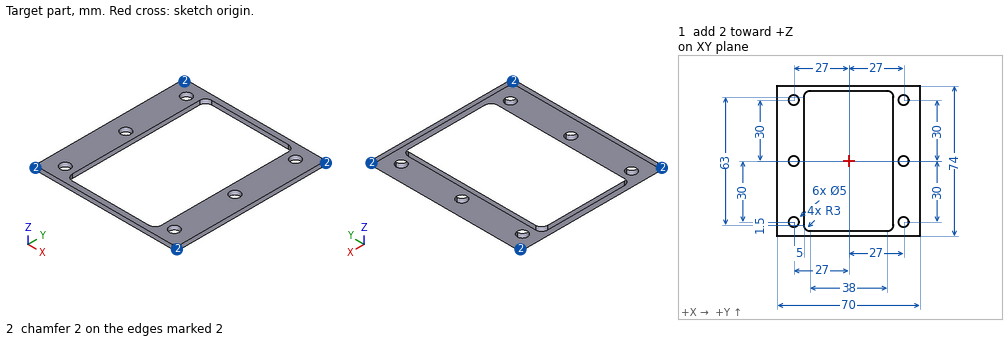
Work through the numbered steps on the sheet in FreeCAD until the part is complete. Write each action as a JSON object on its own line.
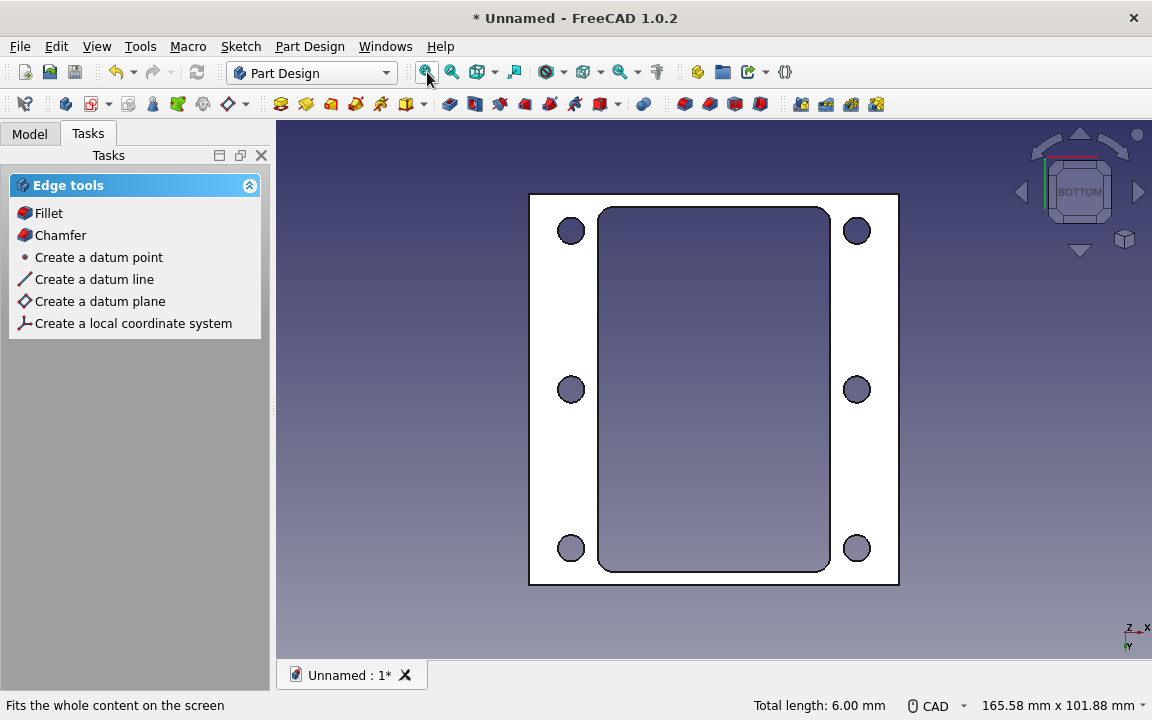
{"action": "scroll", "coordinate": [529, 584], "scroll_direction": "up", "scroll_amount": 7}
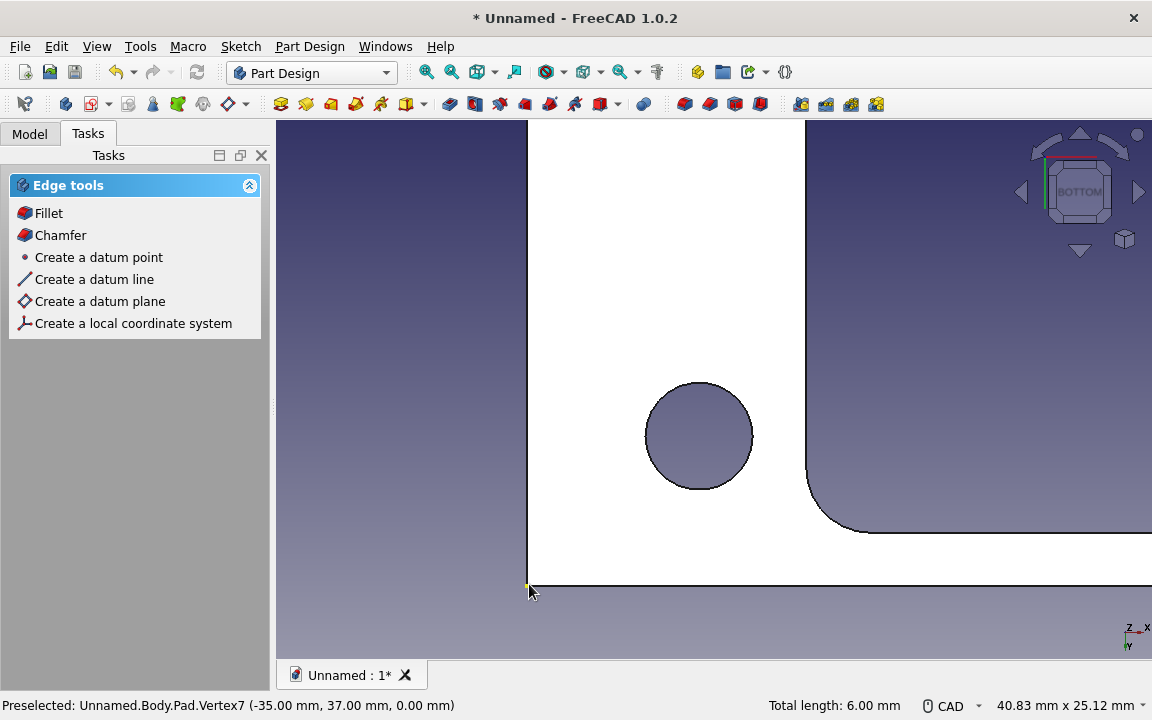
{"action": "left_click", "coordinate": [427, 72]}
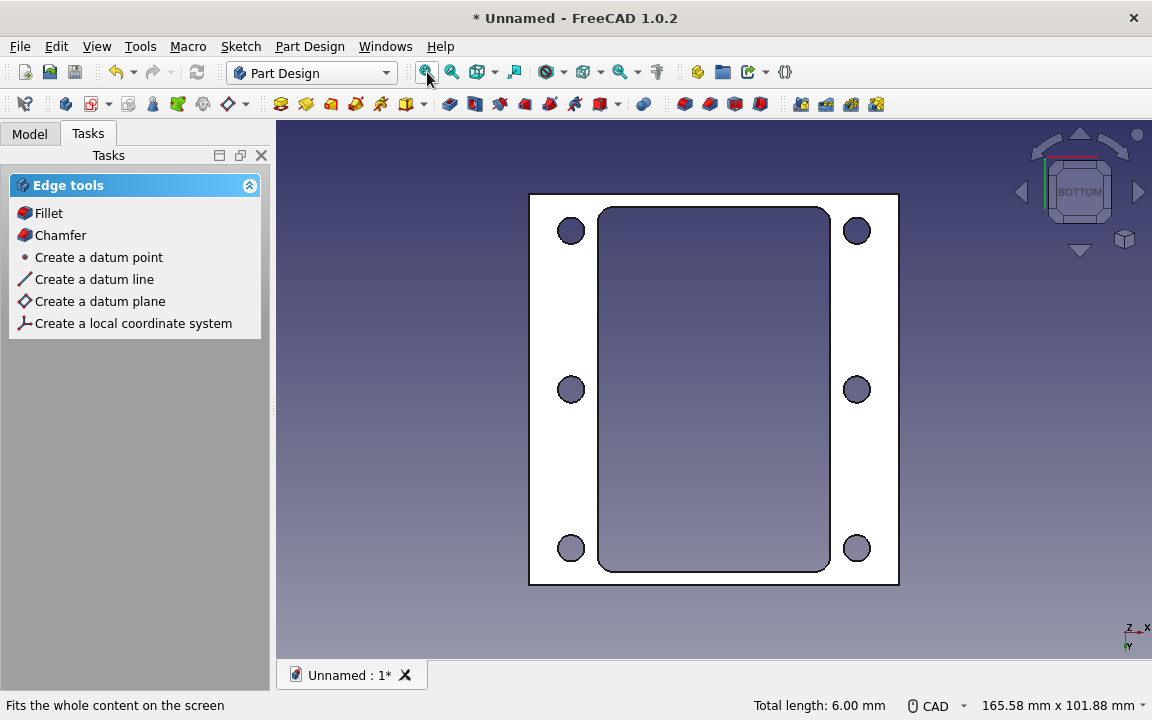
{"action": "key", "text": "4"}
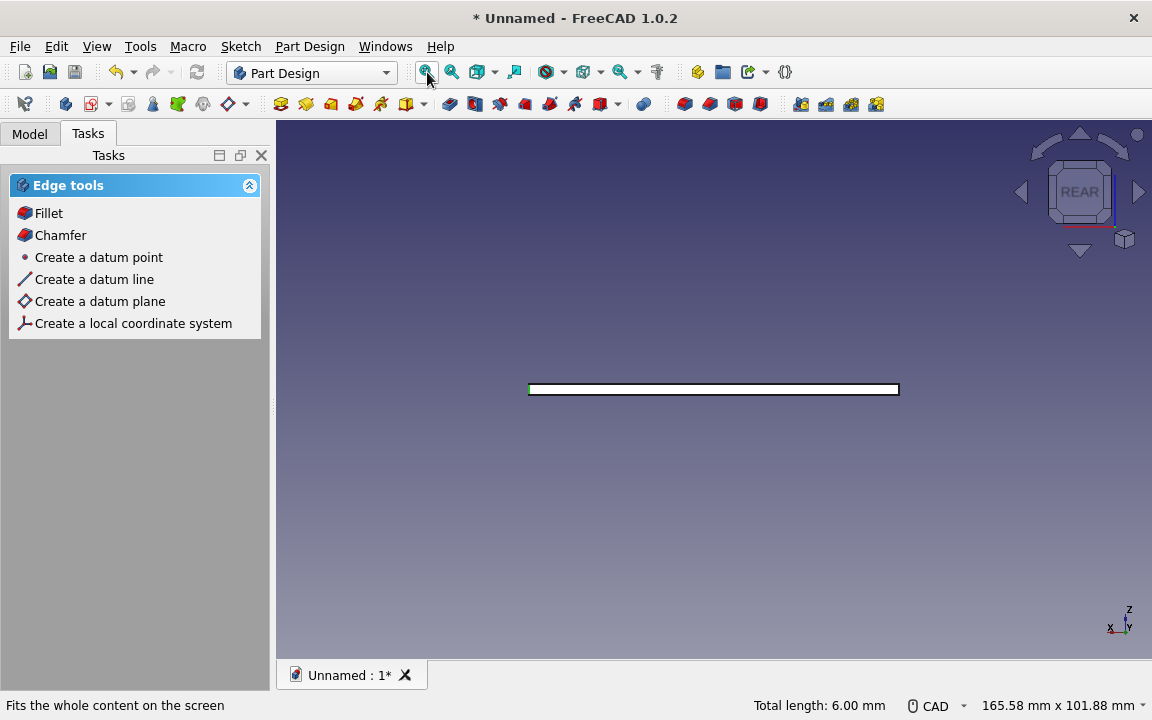
{"action": "left_click", "coordinate": [427, 72]}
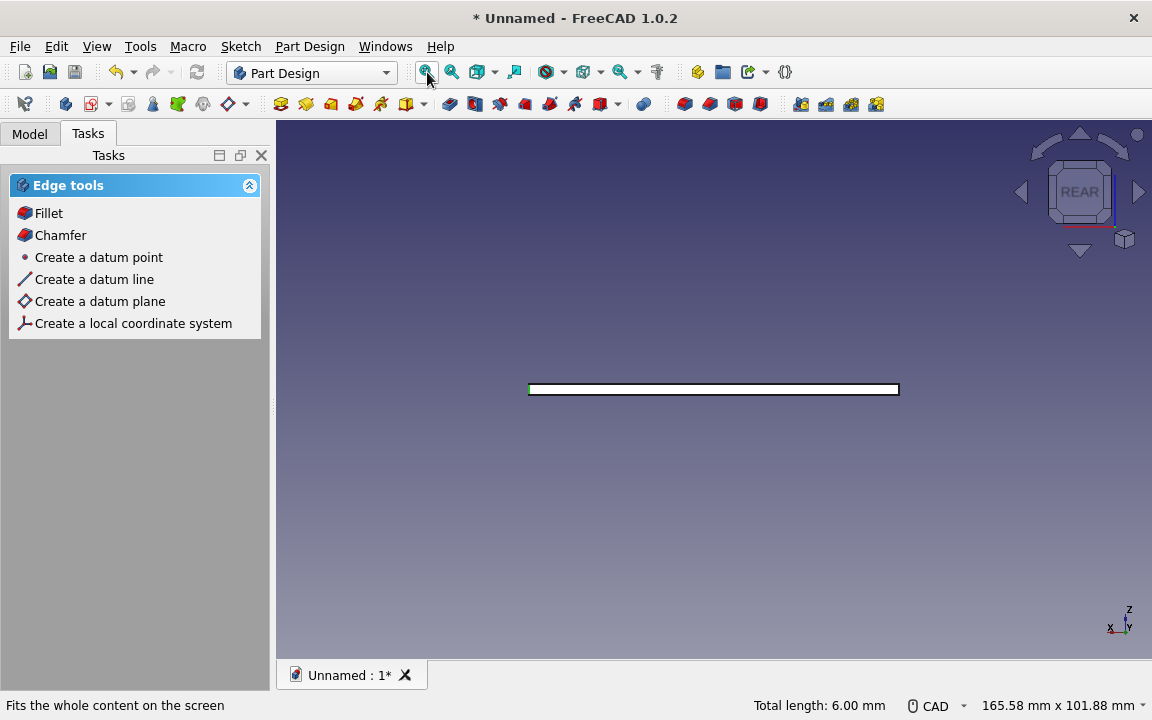
{"action": "scroll", "coordinate": [899, 389], "scroll_direction": "up", "scroll_amount": 7}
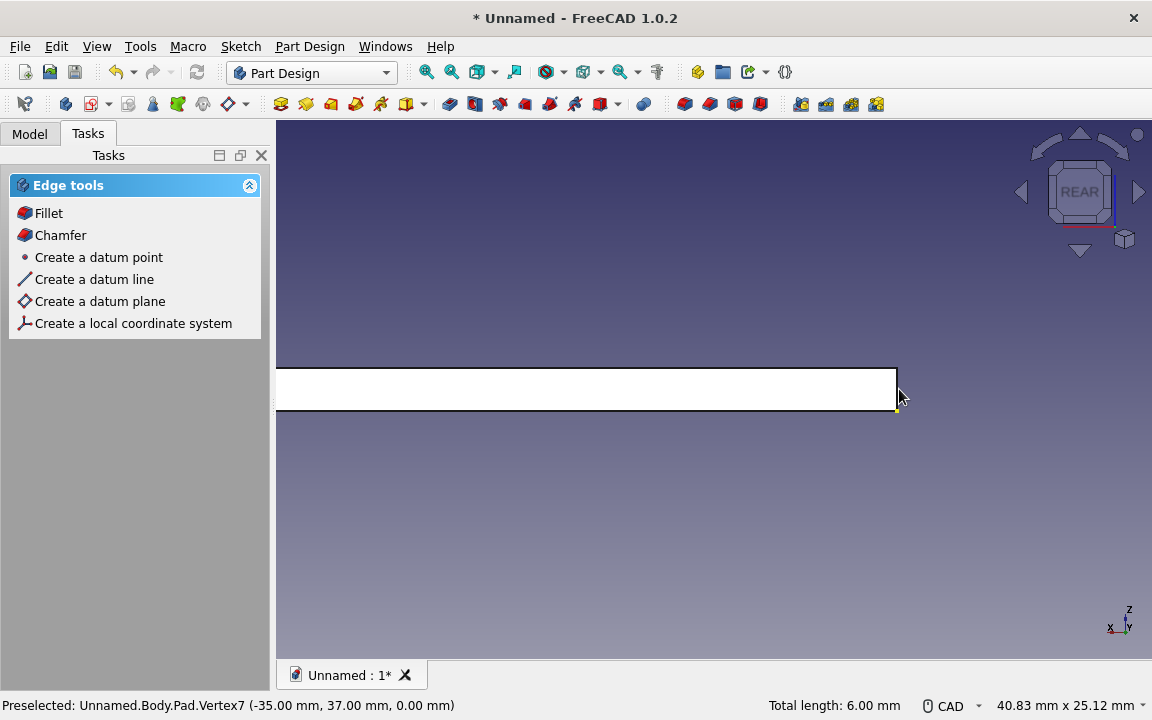
{"action": "left_click", "coordinate": [897, 389], "text": "ctrl"}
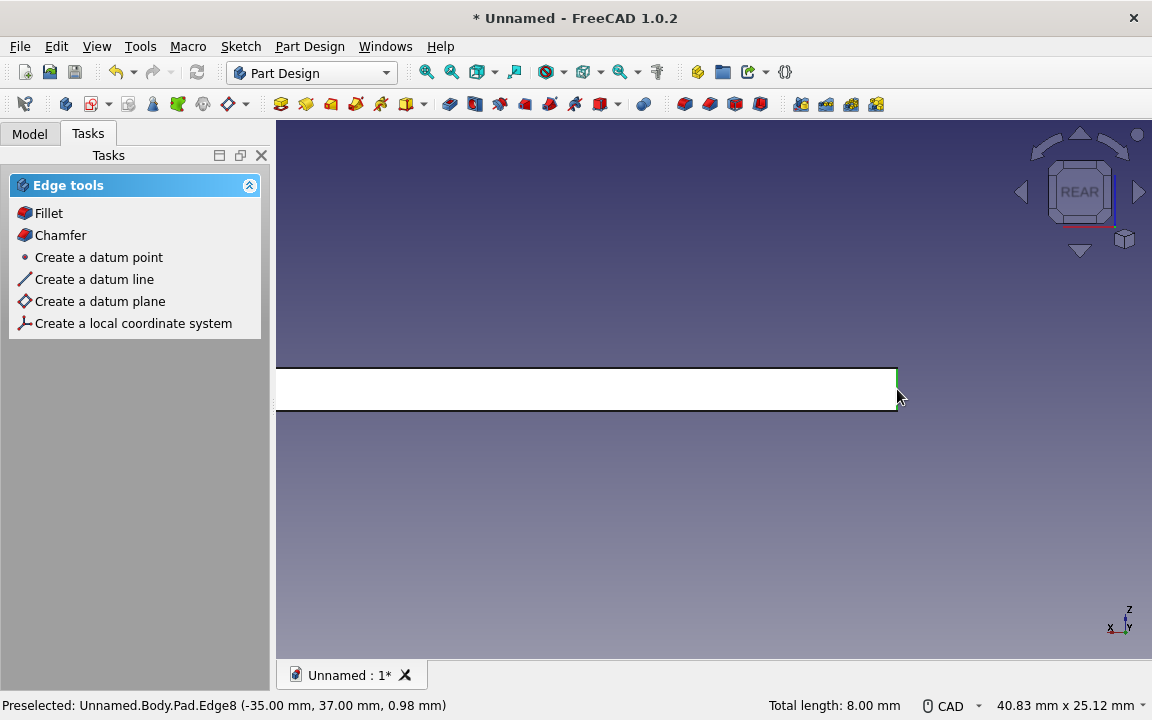
{"action": "left_click", "coordinate": [710, 104]}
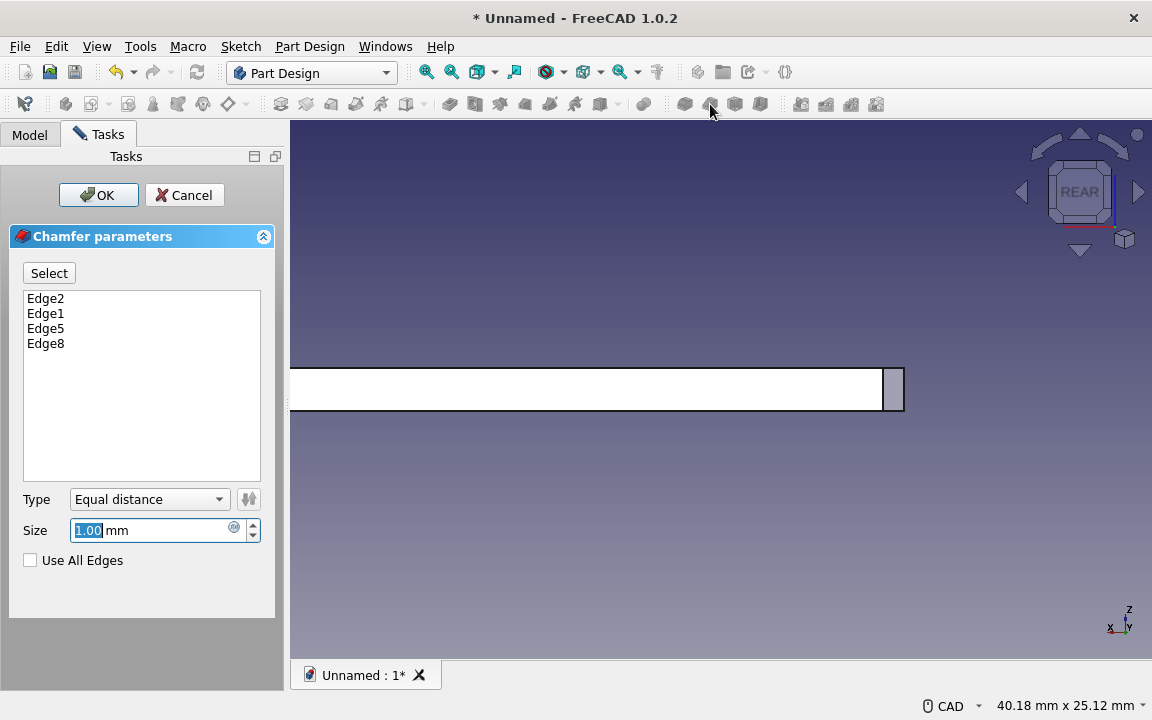
{"action": "type", "text": "2"}
{"action": "key", "text": "Tab"}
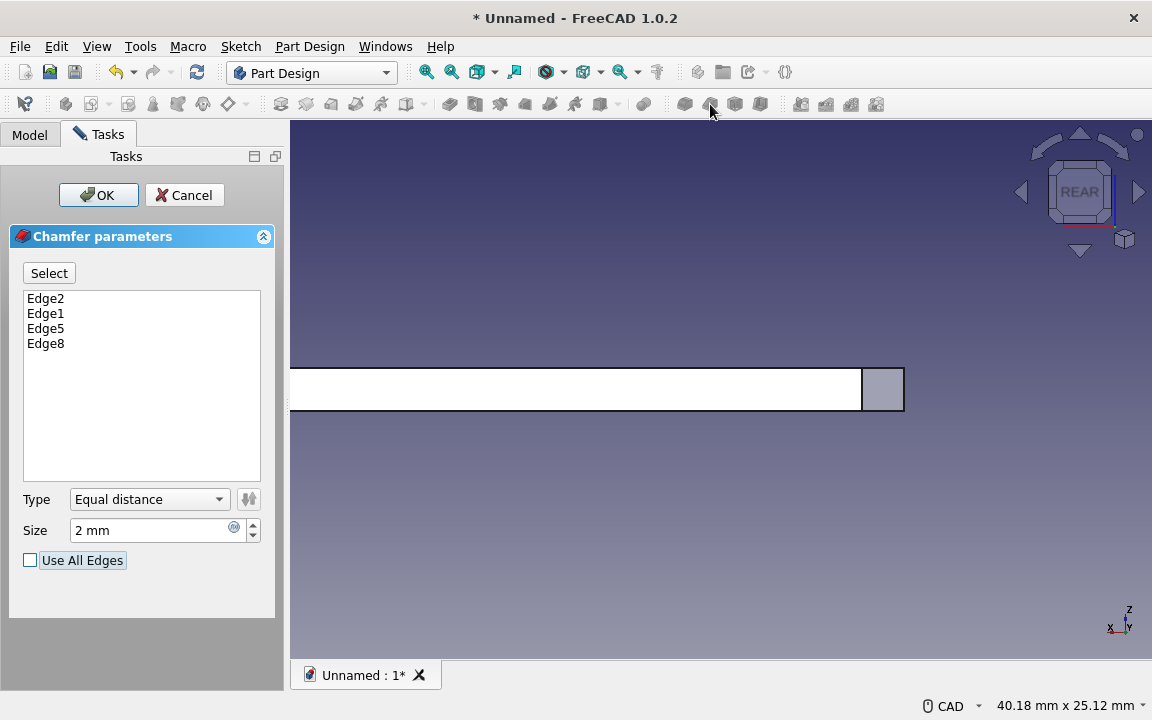
{"action": "left_click", "coordinate": [99, 195]}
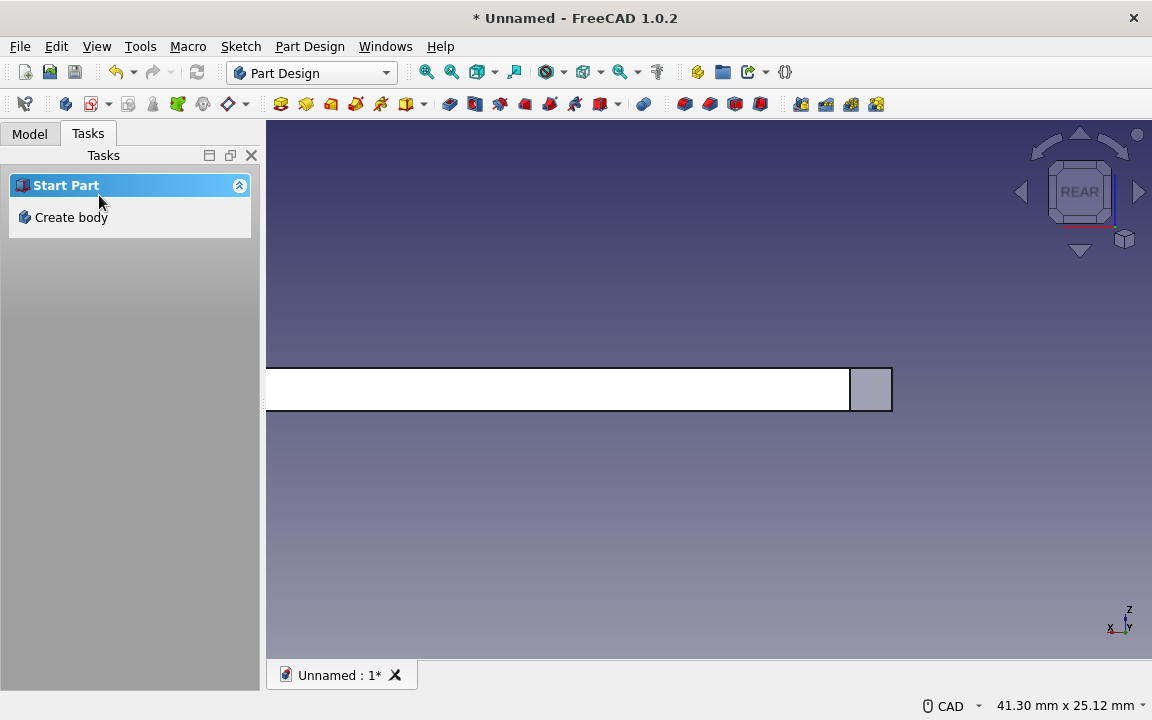
{"action": "key", "text": "0"}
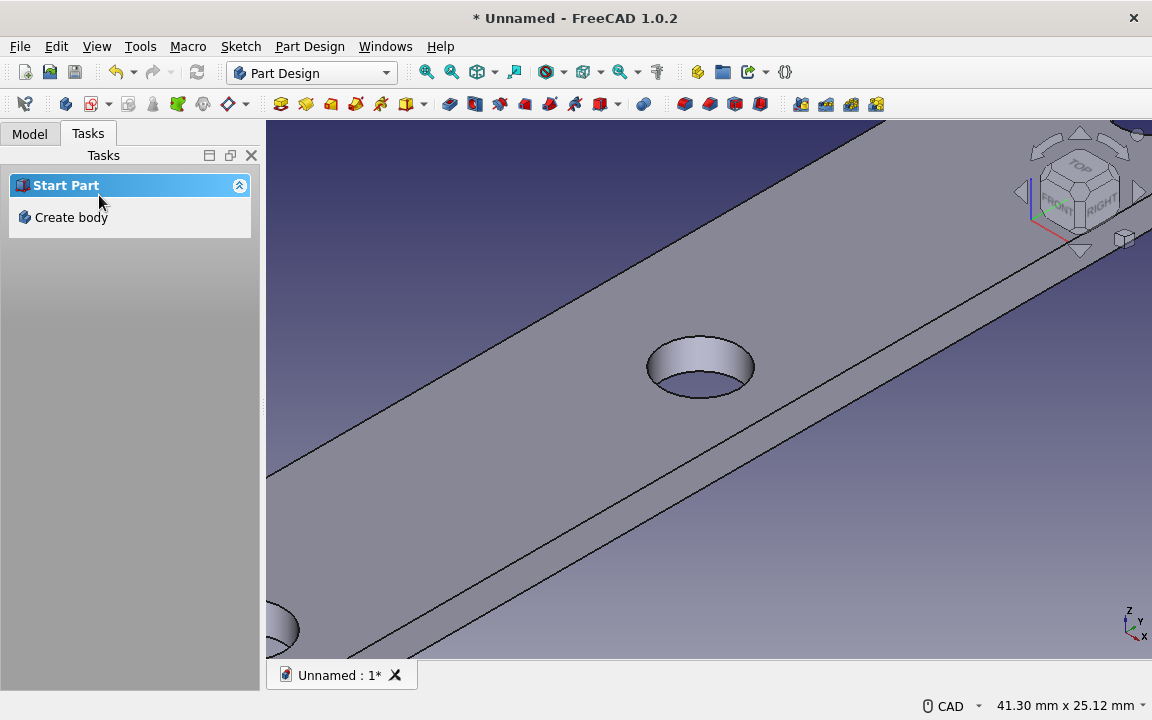
{"action": "left_click", "coordinate": [427, 72]}